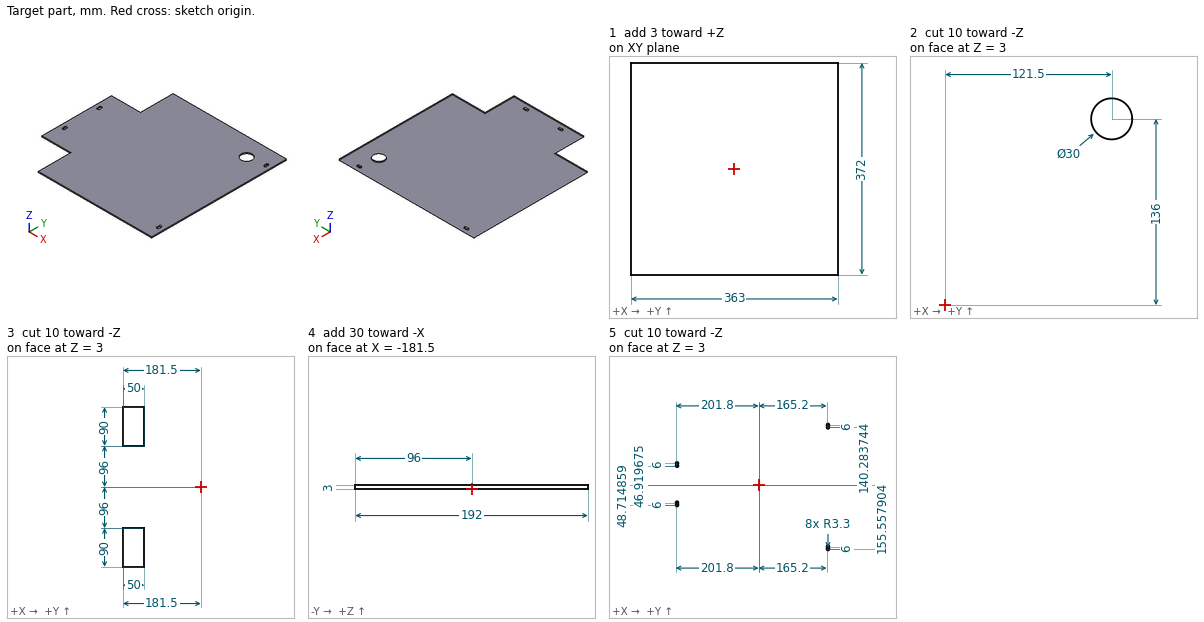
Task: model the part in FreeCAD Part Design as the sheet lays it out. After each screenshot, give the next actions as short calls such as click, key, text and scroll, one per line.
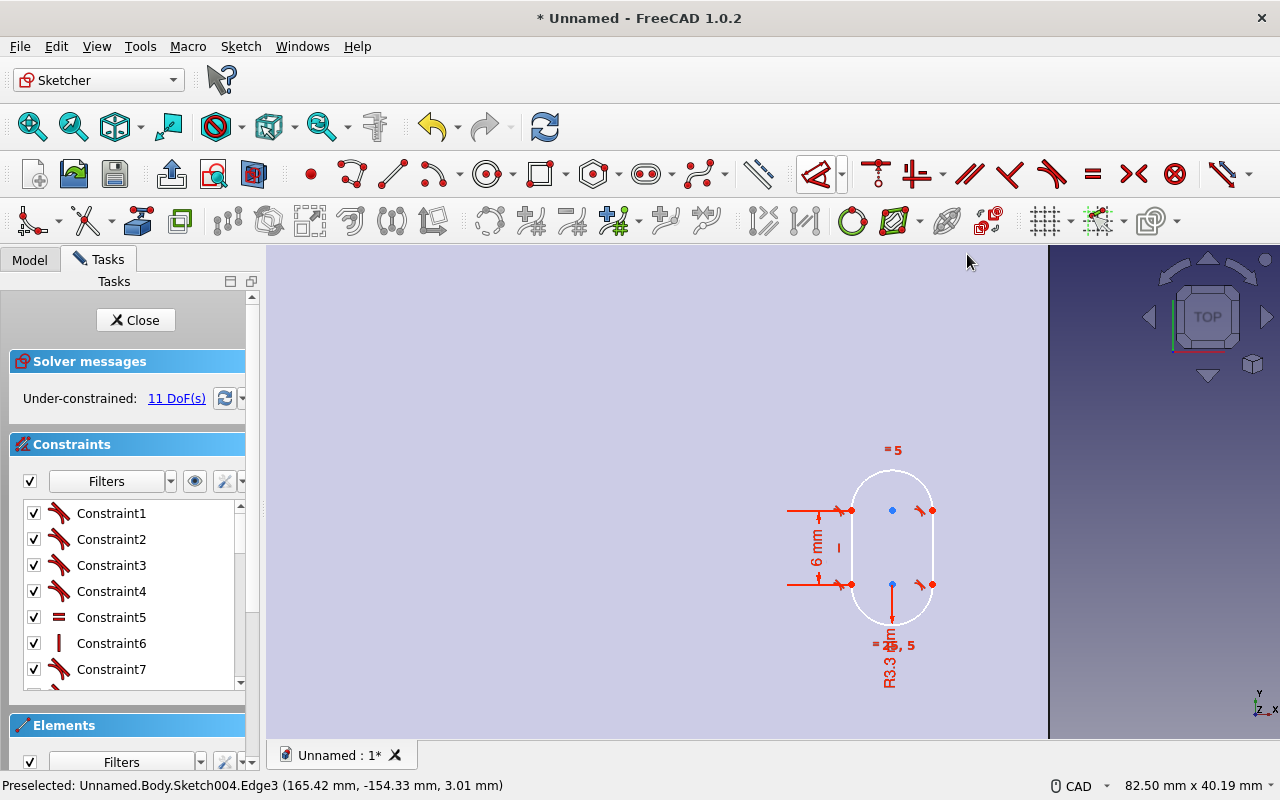
scroll(871, 634, down, 13)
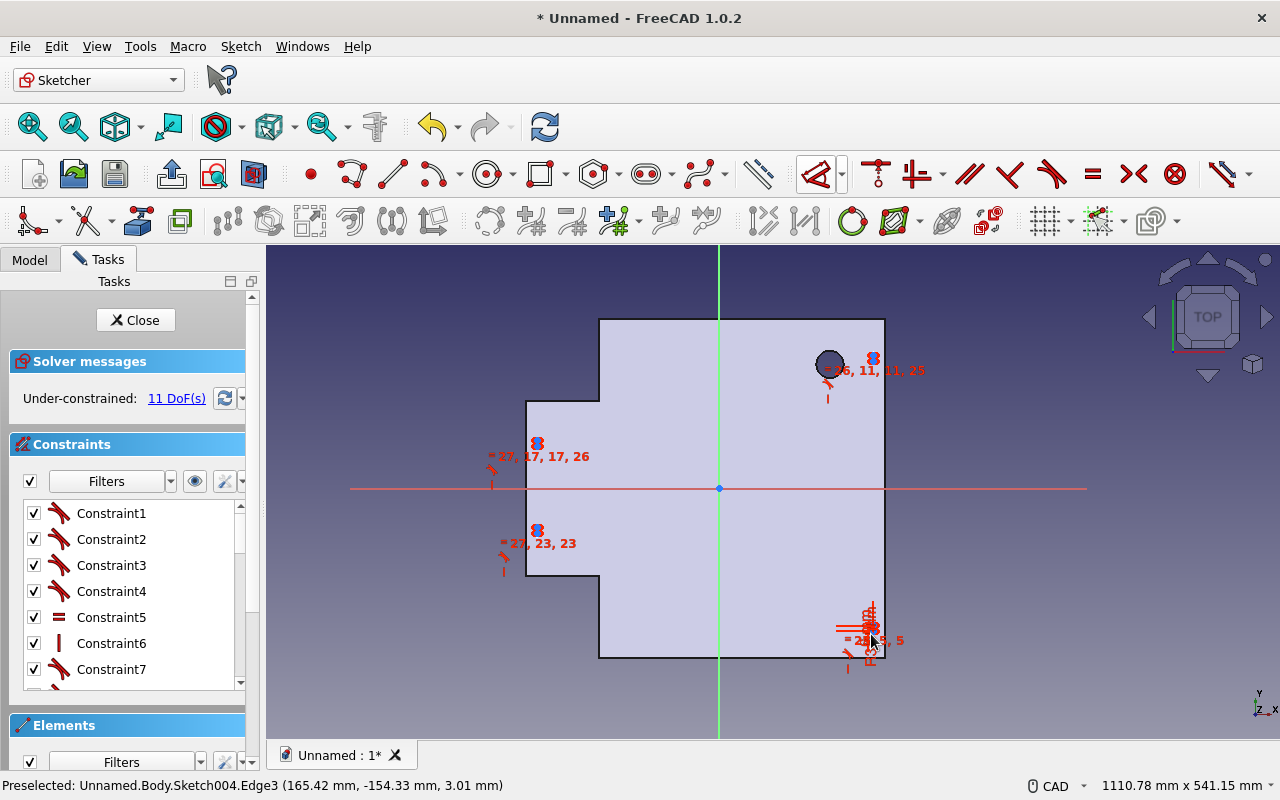
scroll(870, 359, up, 11)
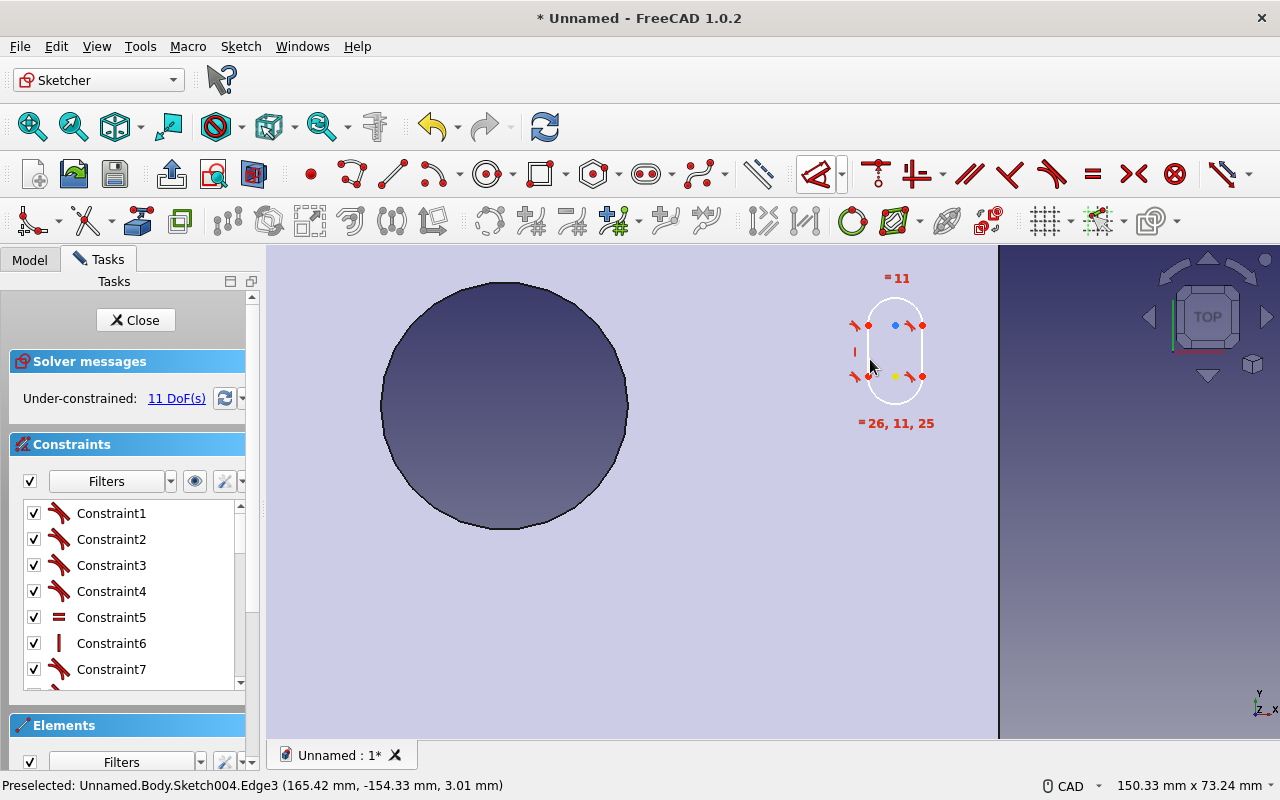
click(868, 361)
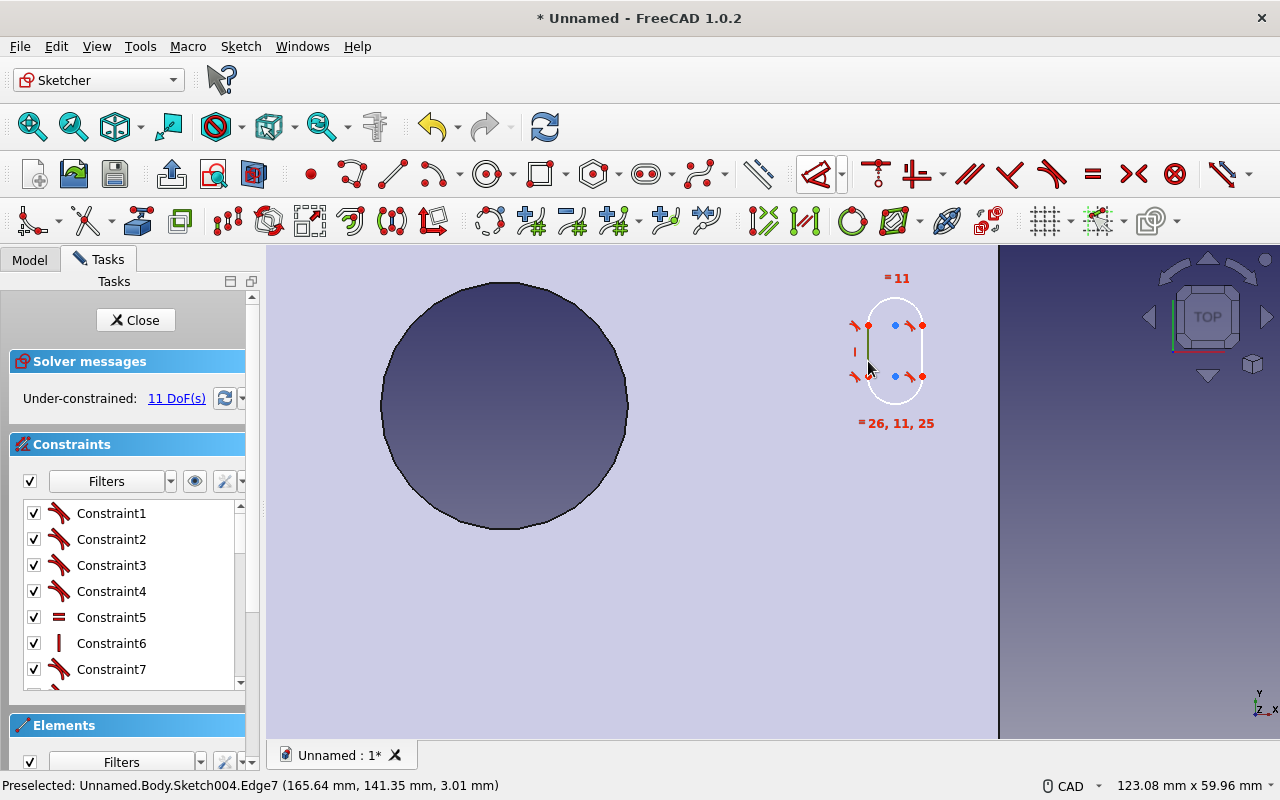
key(i)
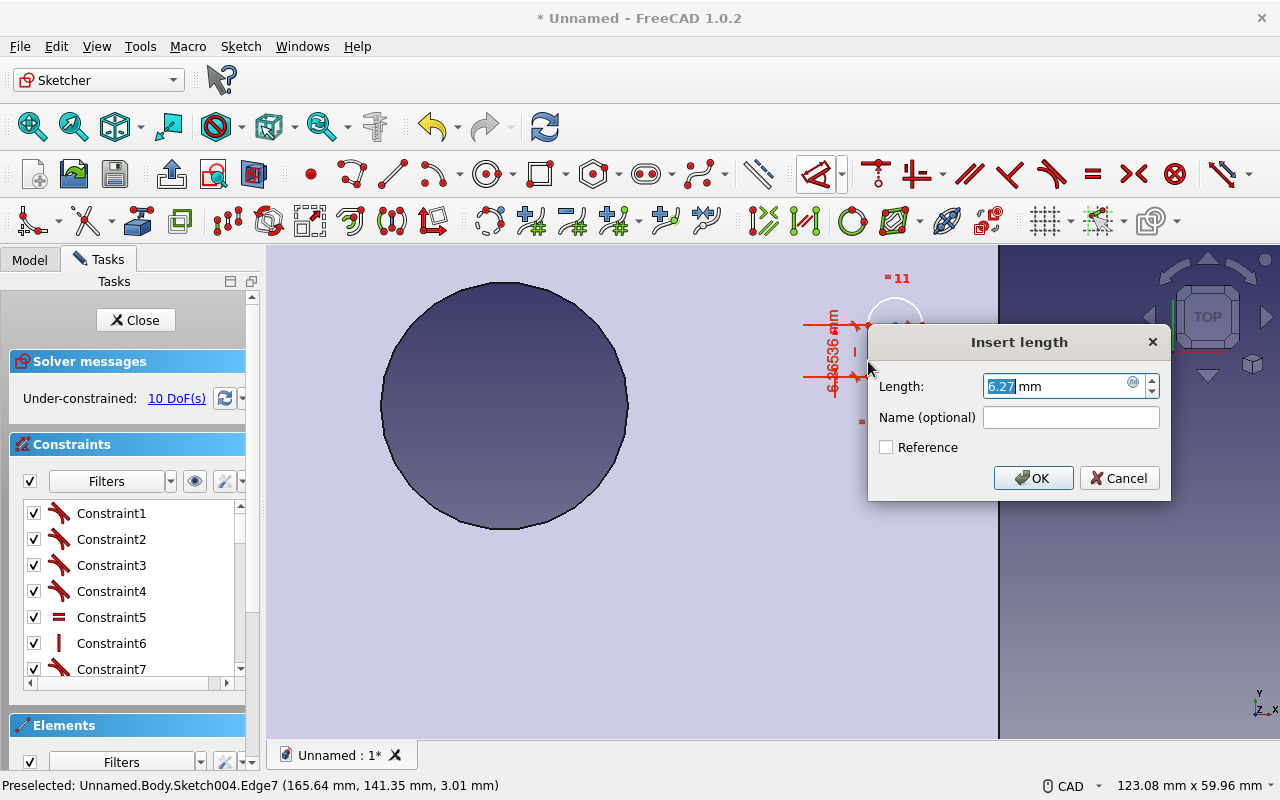
text(6)
key(Return)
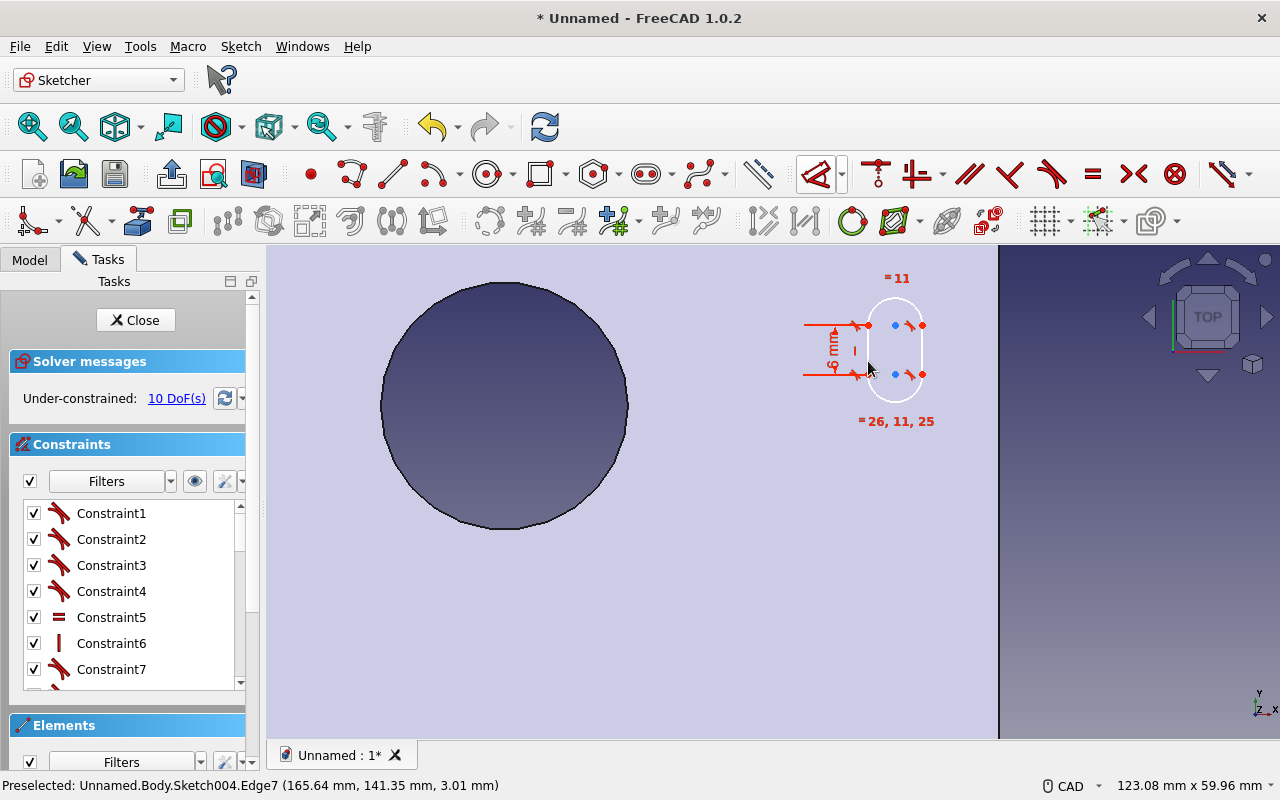
scroll(870, 358, down, 11)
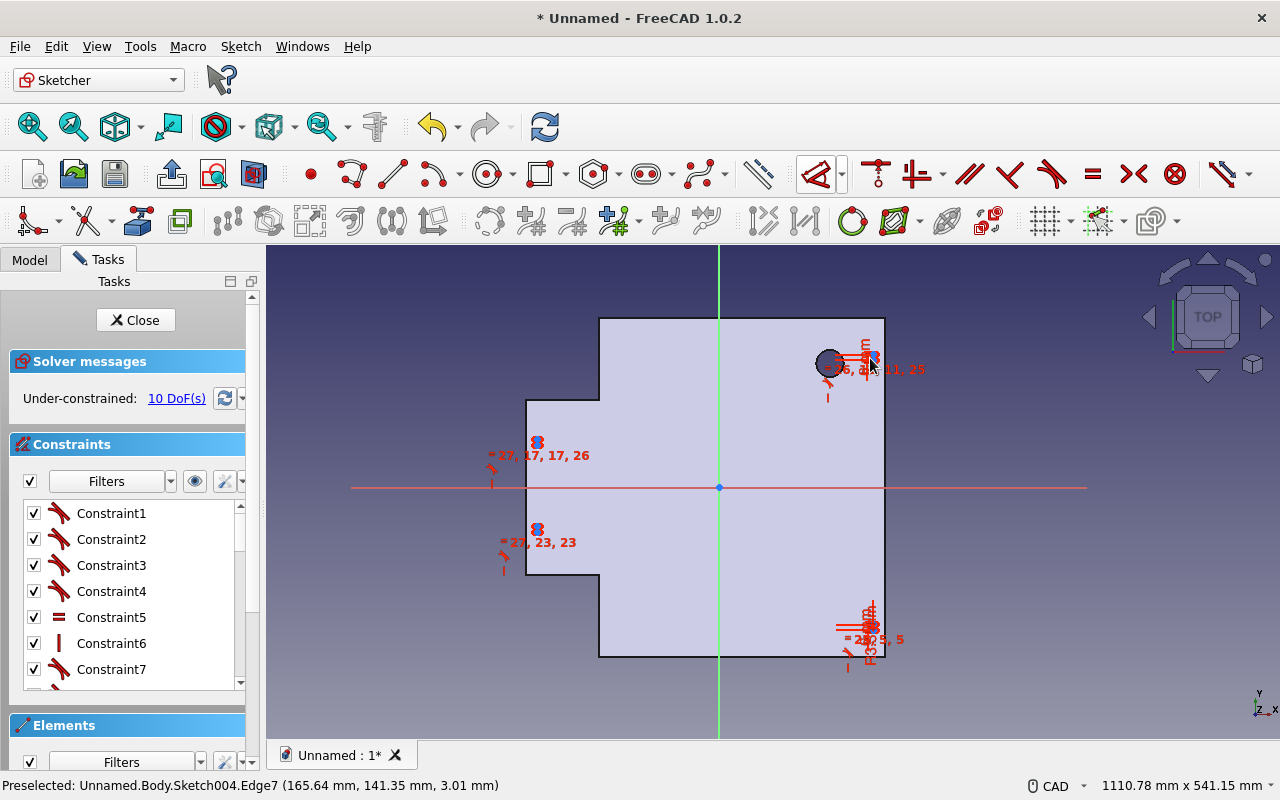
scroll(535, 444, up, 11)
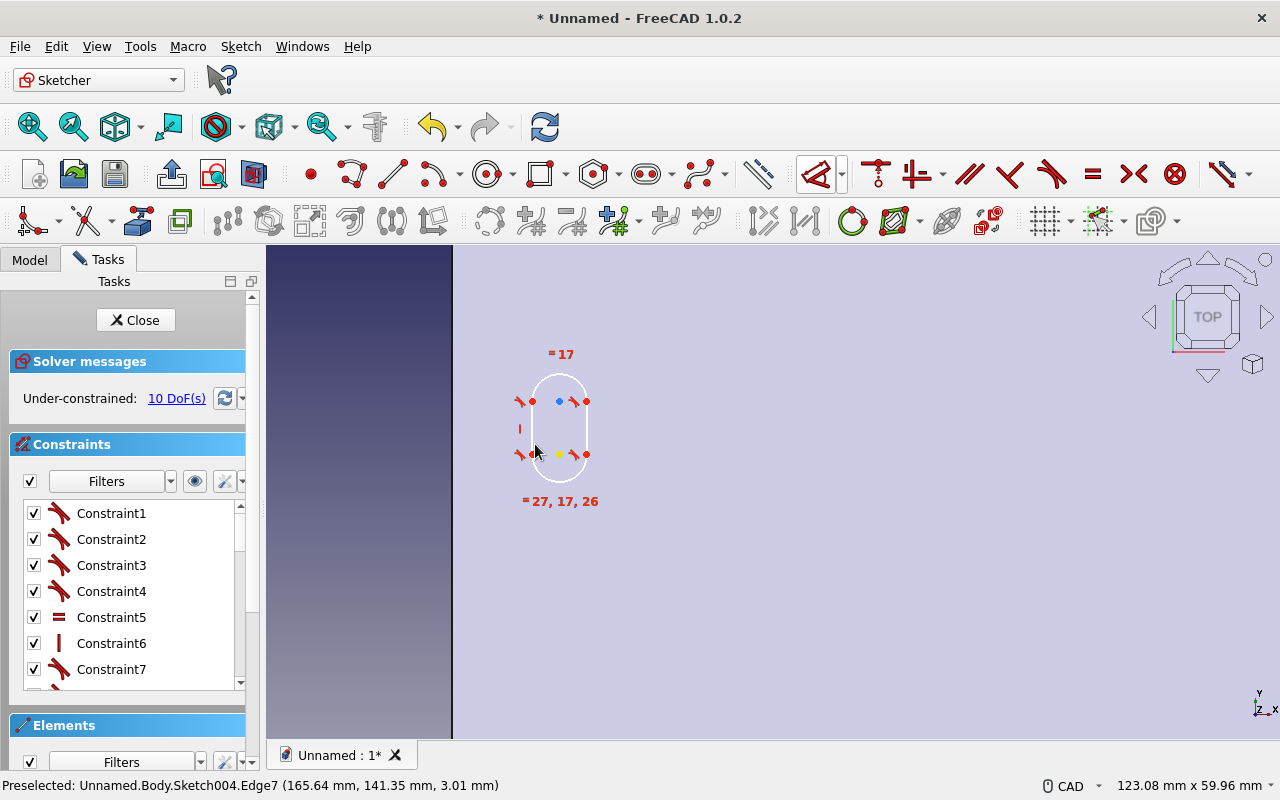
click(532, 439)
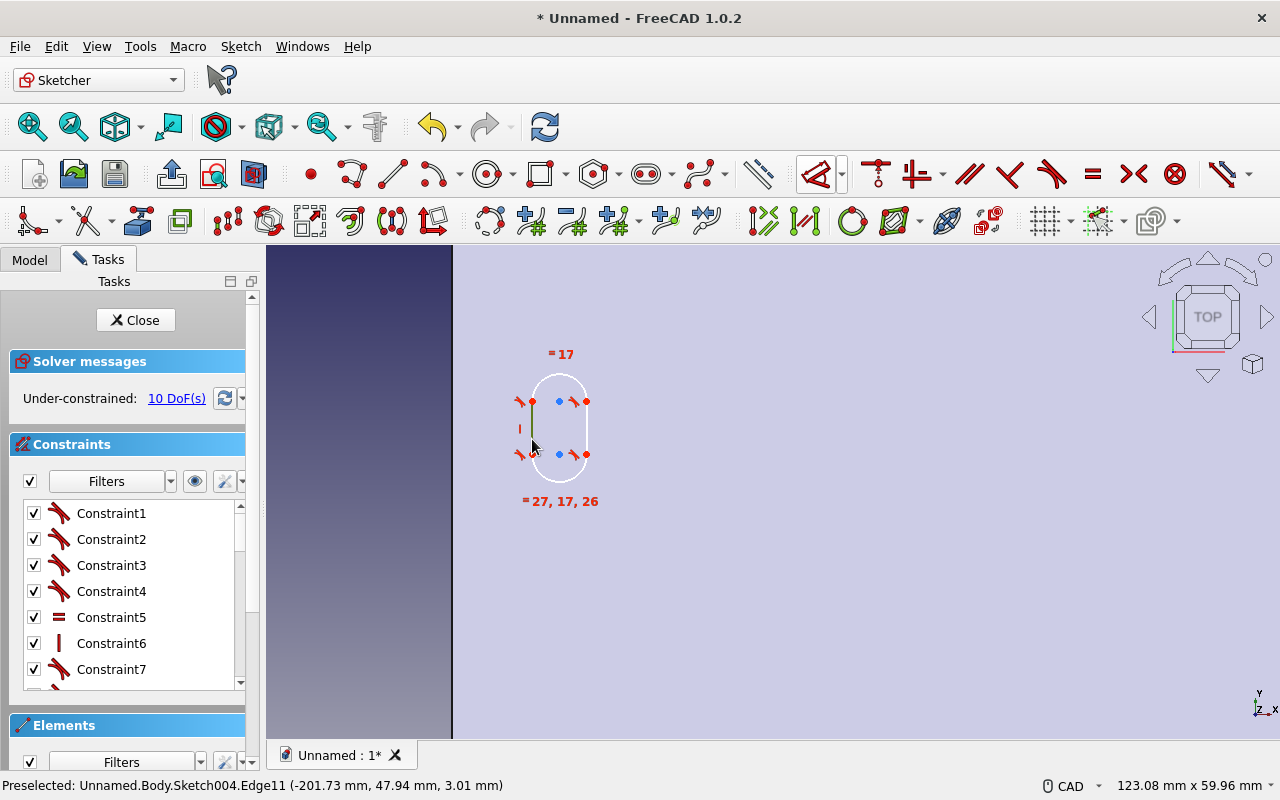
click(842, 174)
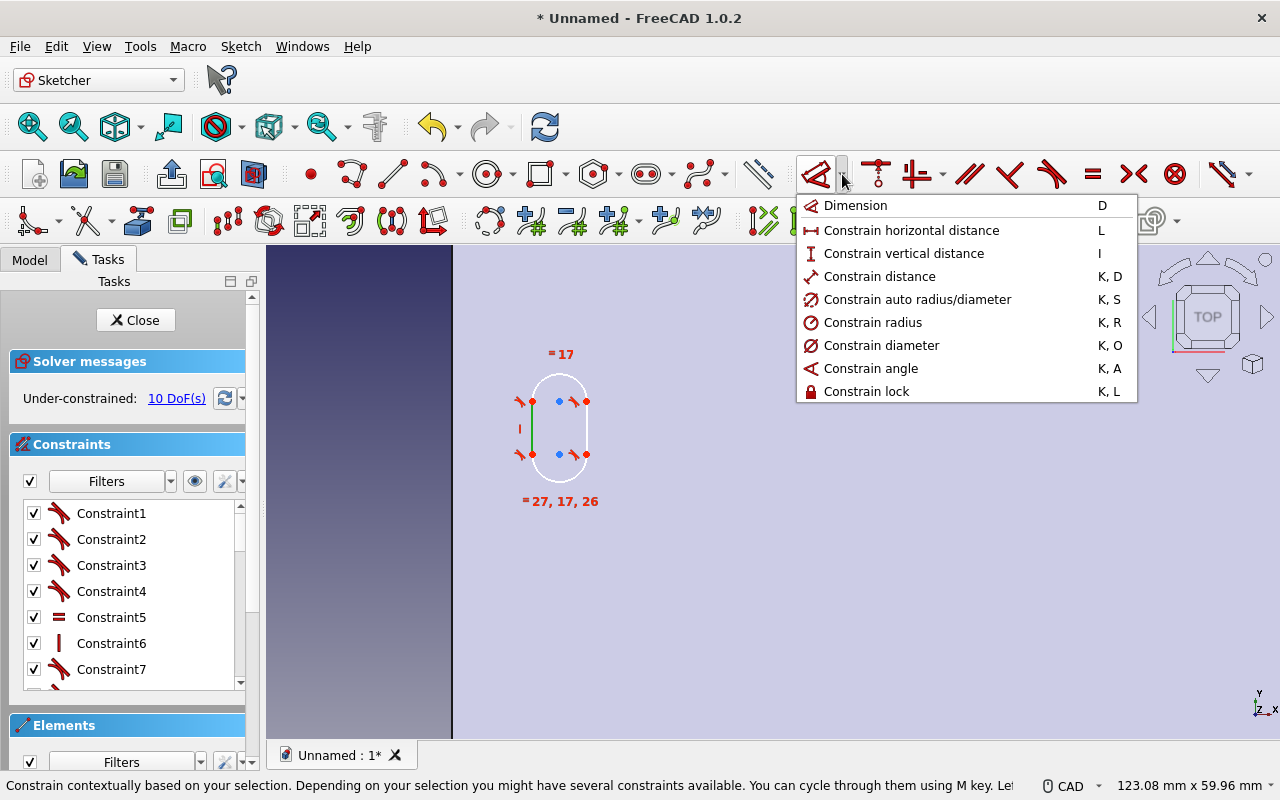
click(967, 254)